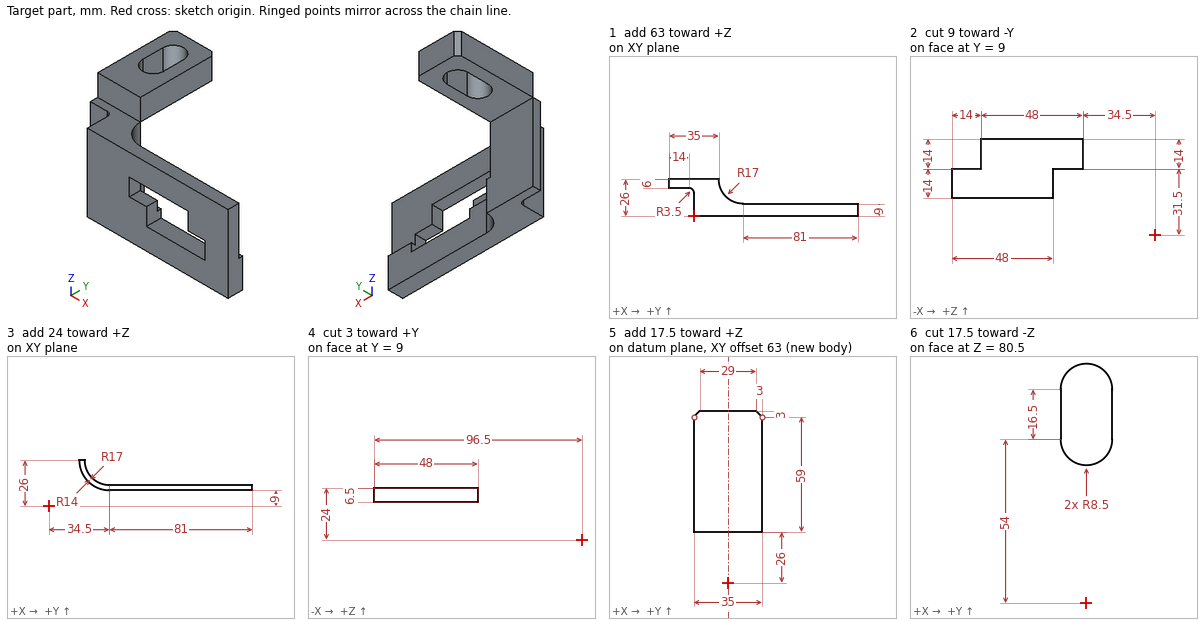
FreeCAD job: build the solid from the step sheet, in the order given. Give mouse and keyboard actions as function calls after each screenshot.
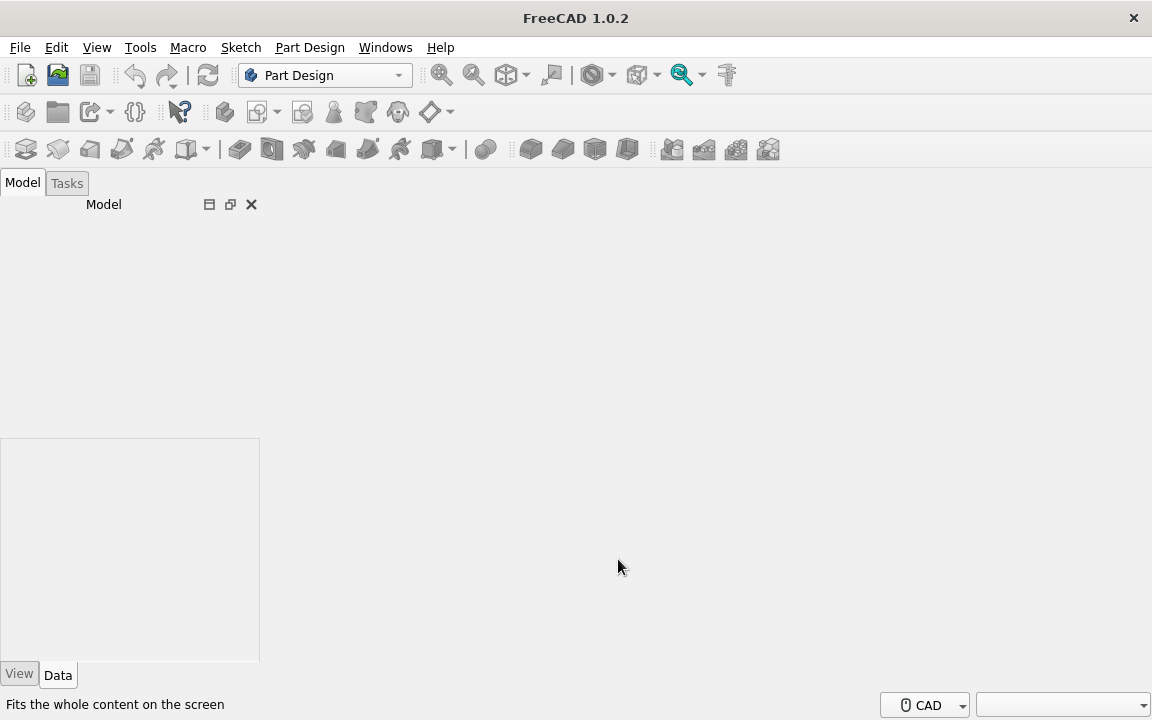
key(ctrl+n)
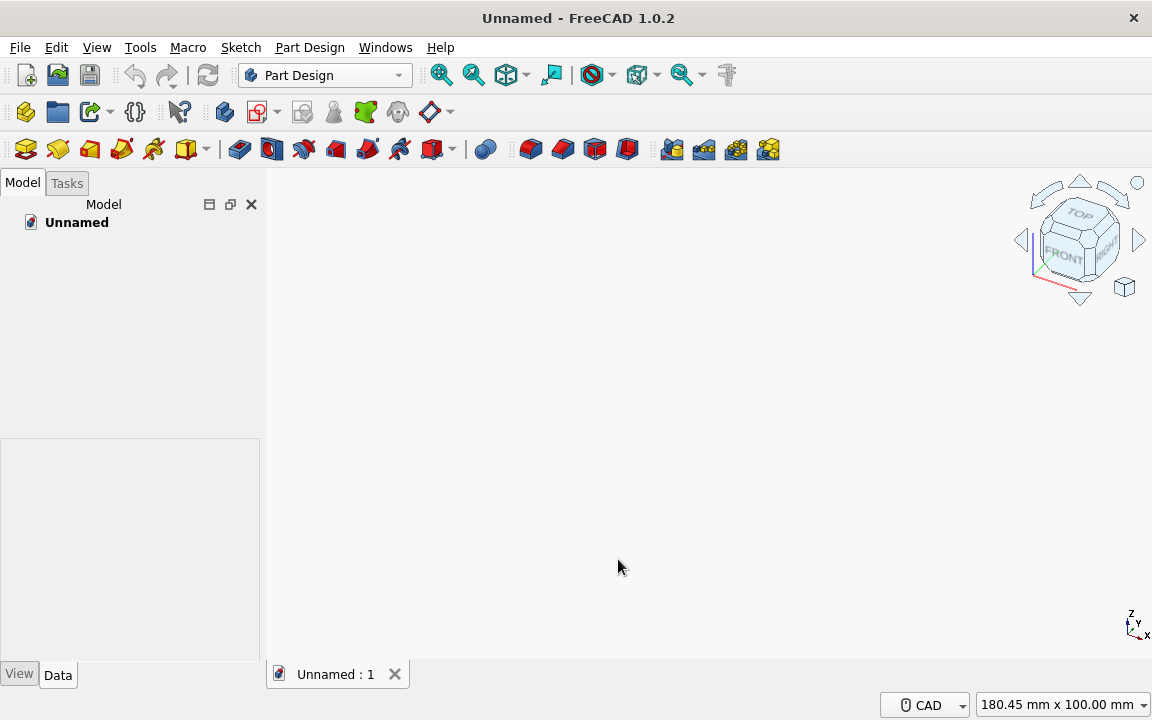
click(258, 112)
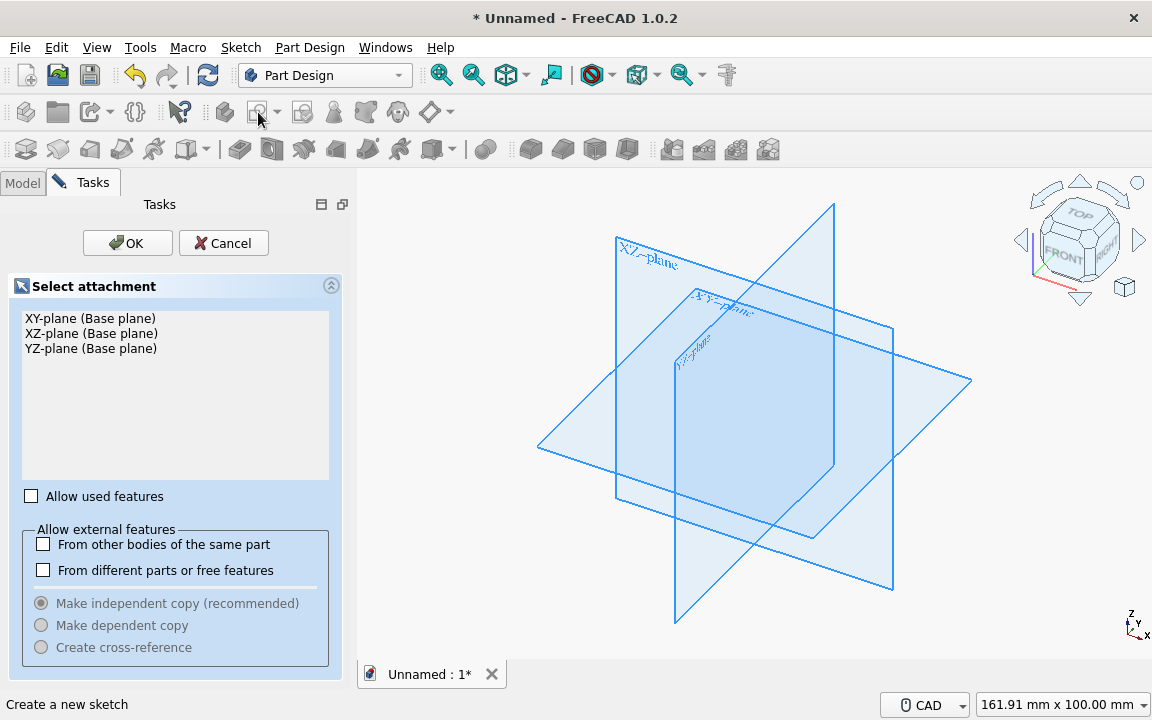
click(82, 318)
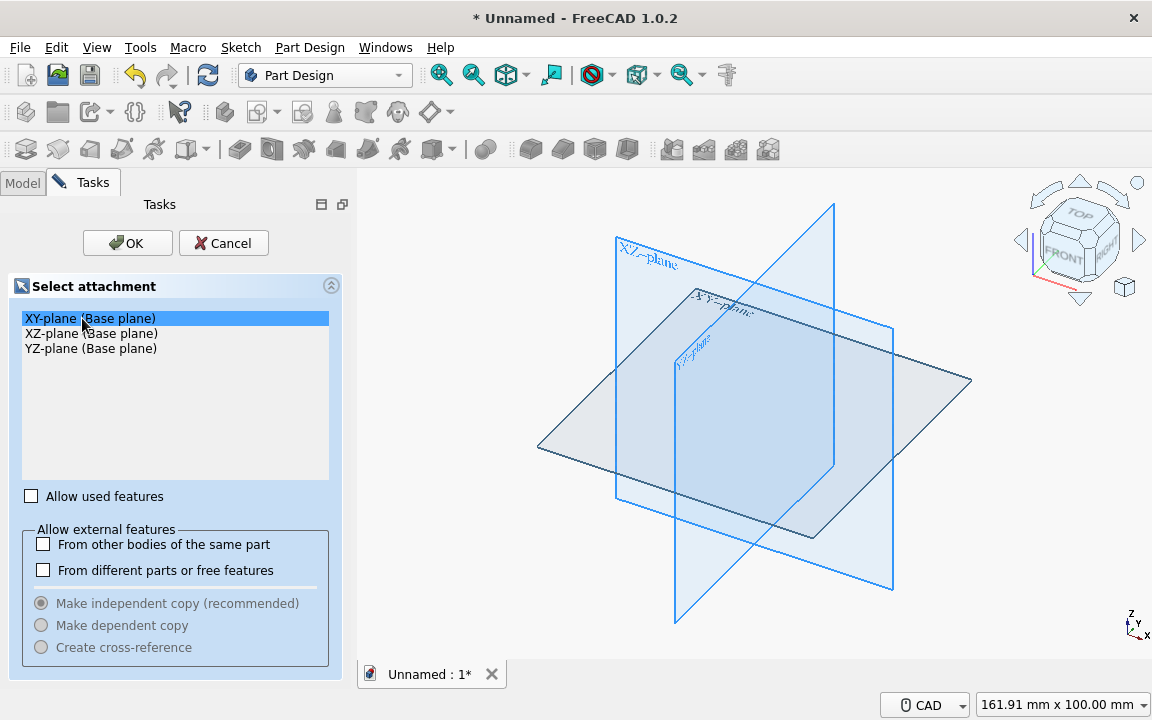
click(128, 243)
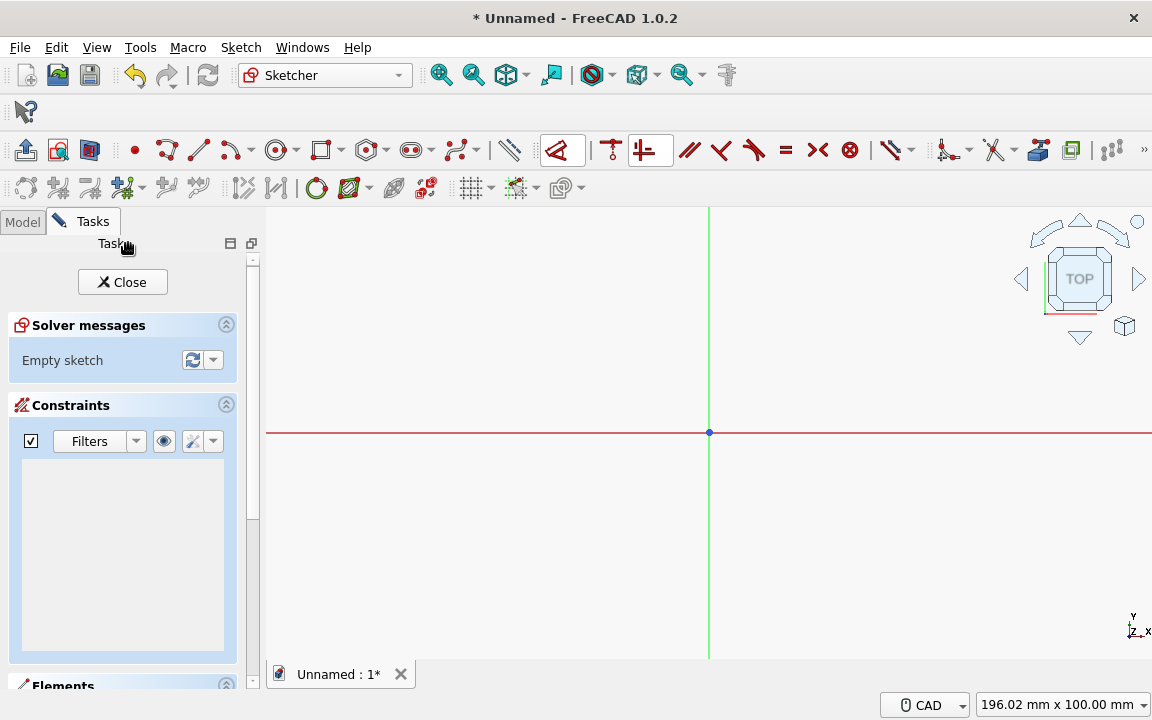
scroll(294, 552, down, 2)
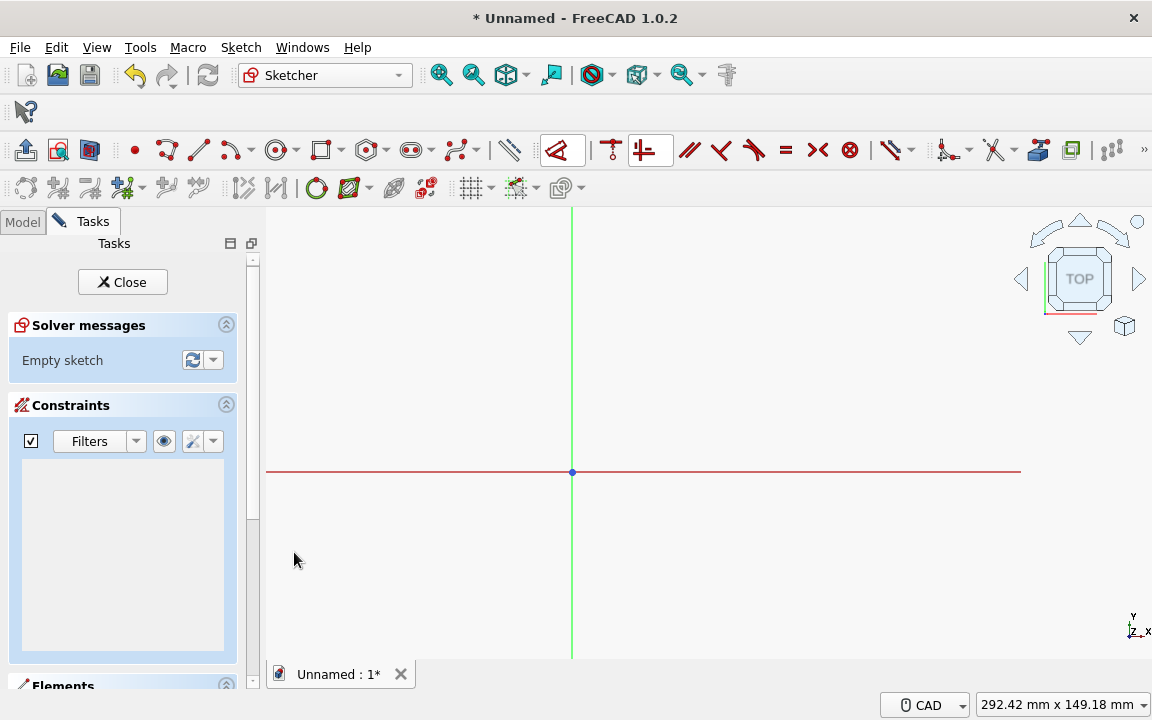
click(168, 150)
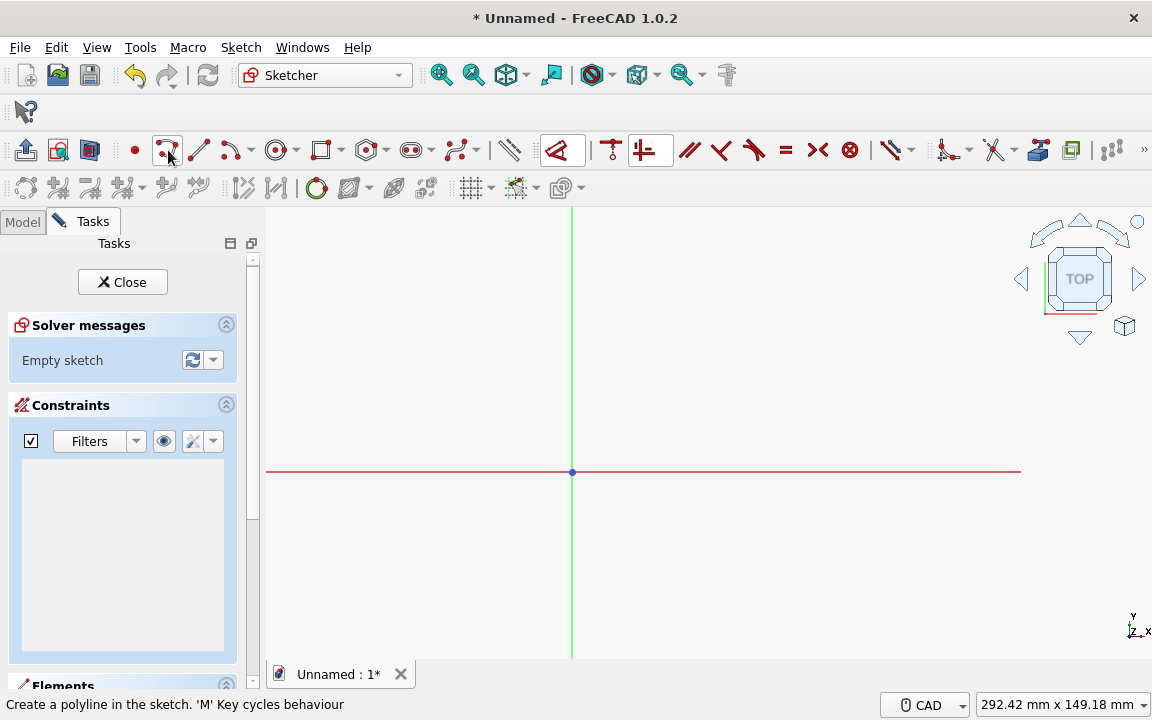
click(625, 394)
click(519, 394)
click(519, 412)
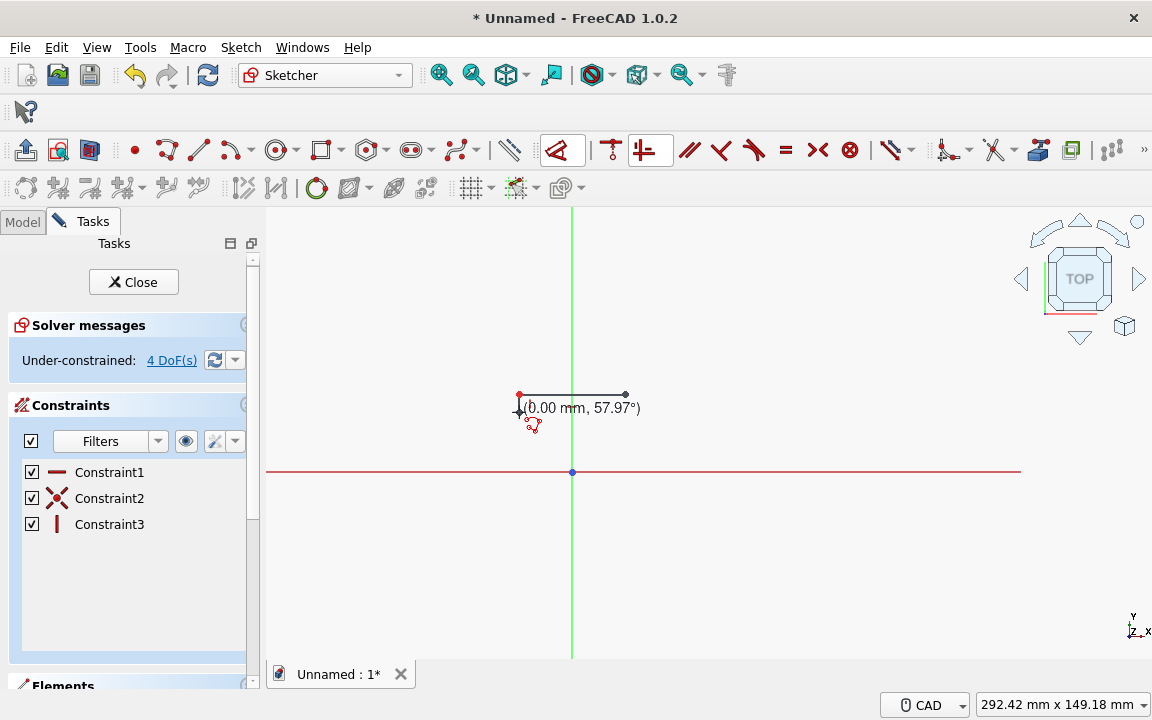
scroll(562, 412, up, 3)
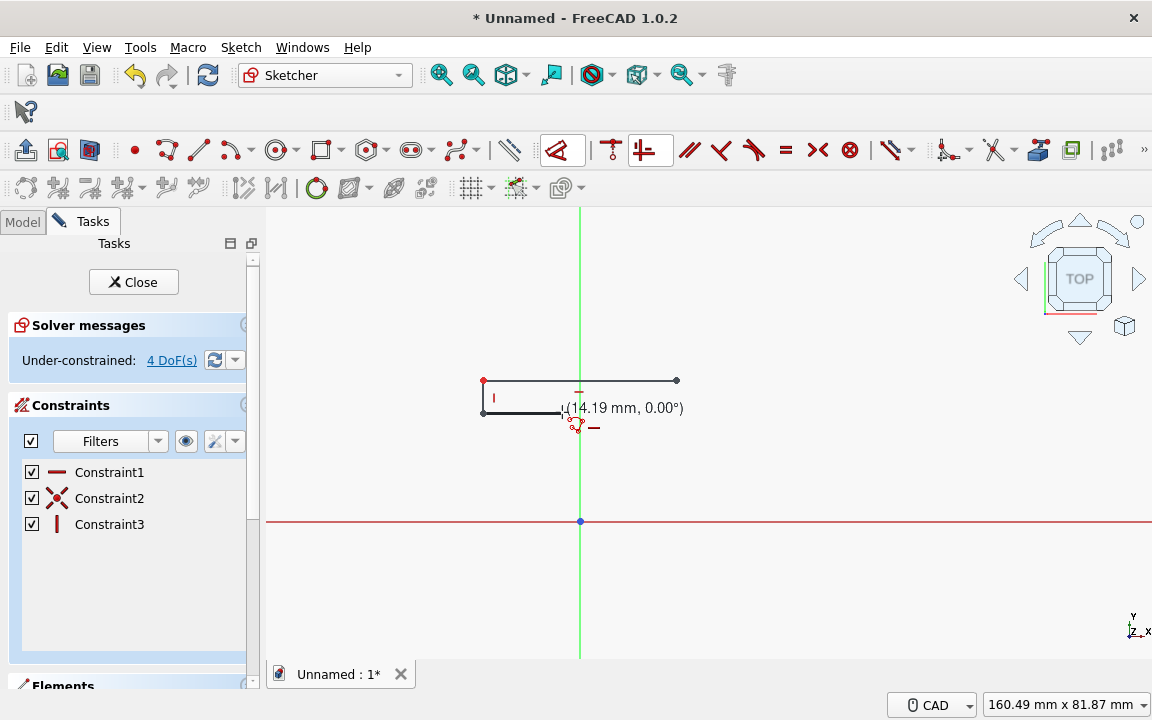
click(561, 412)
right_click(561, 412)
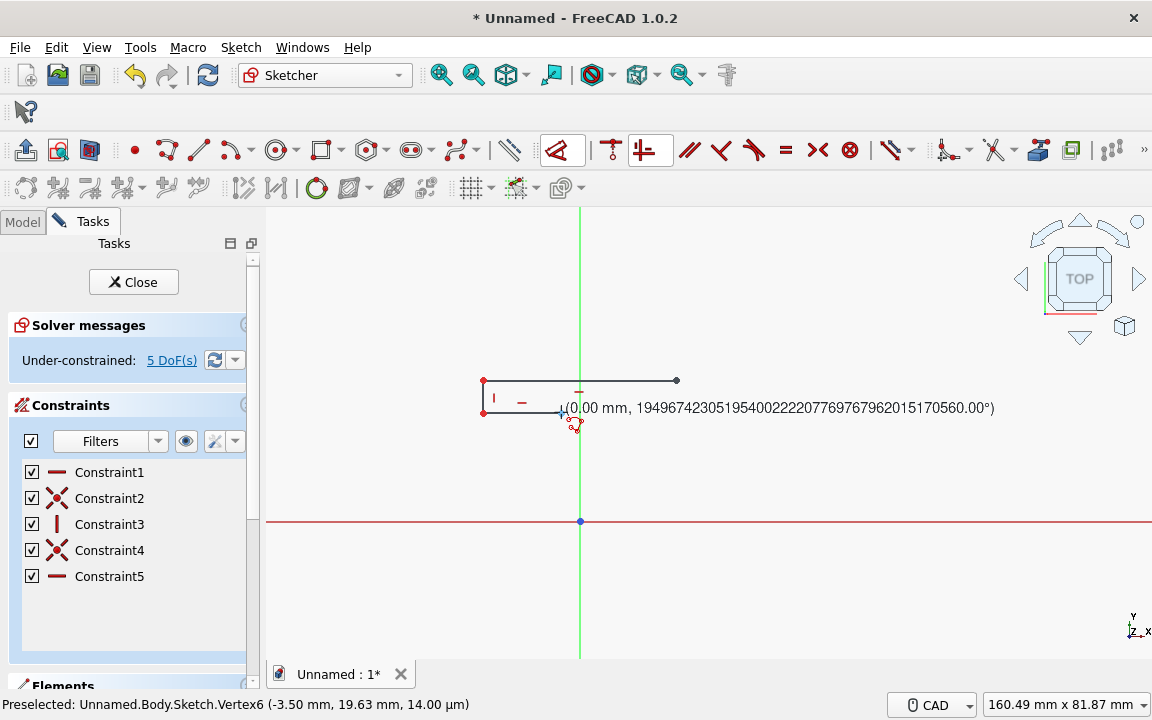
click(580, 431)
click(580, 522)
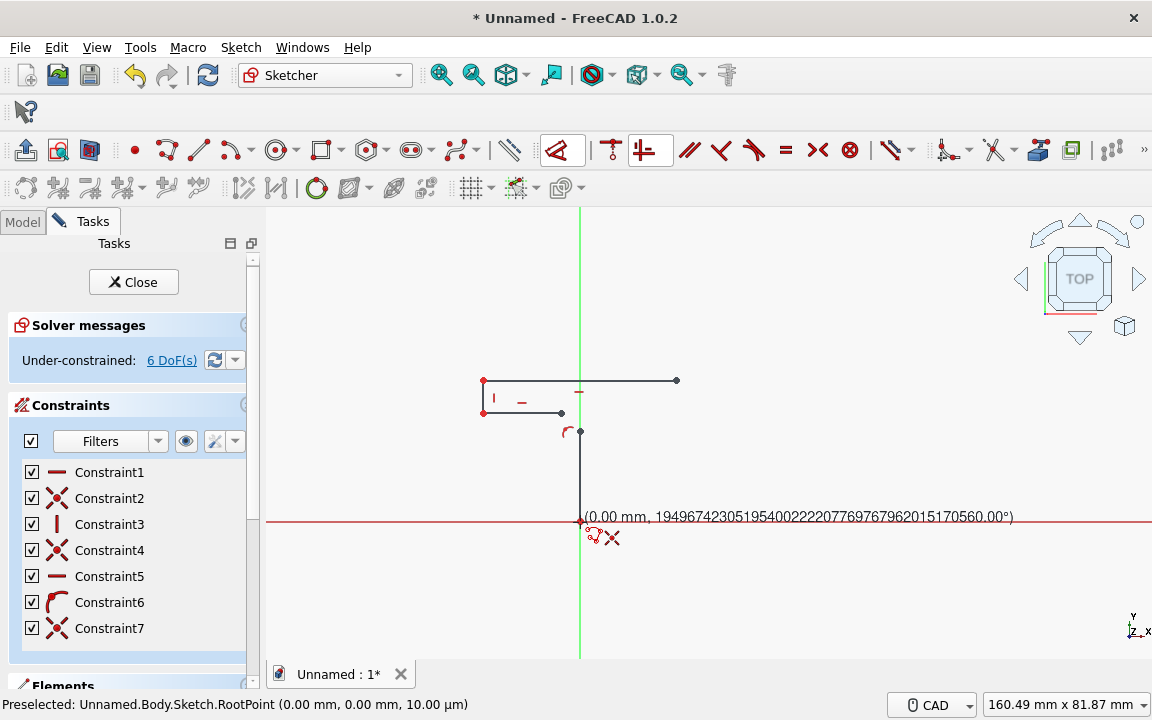
scroll(294, 398, down, 2)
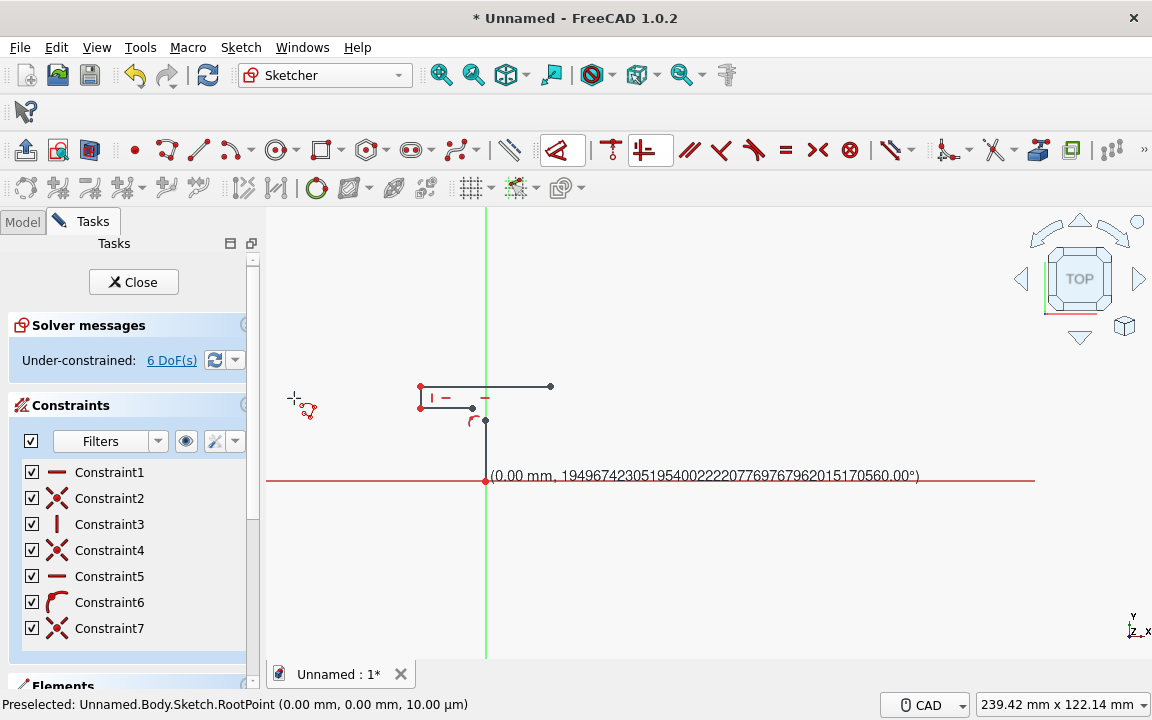
click(913, 472)
click(913, 448)
click(614, 448)
right_click(614, 448)